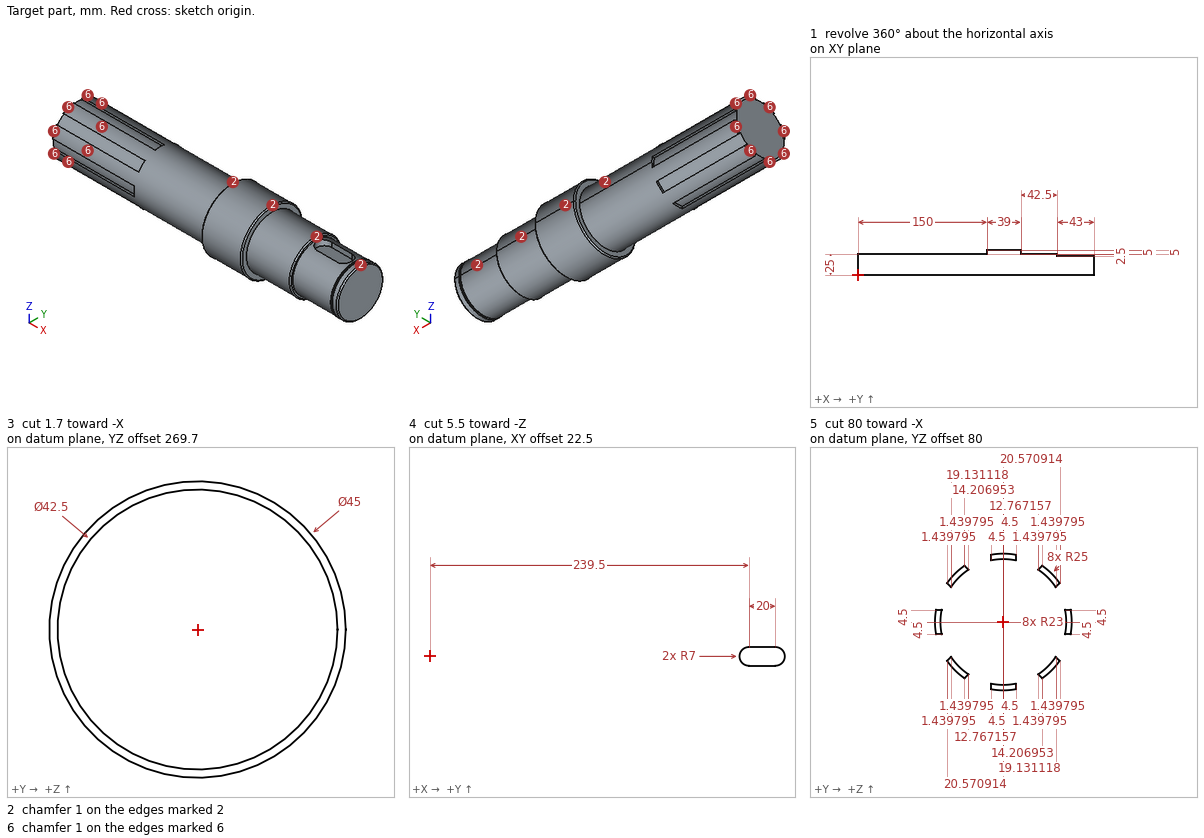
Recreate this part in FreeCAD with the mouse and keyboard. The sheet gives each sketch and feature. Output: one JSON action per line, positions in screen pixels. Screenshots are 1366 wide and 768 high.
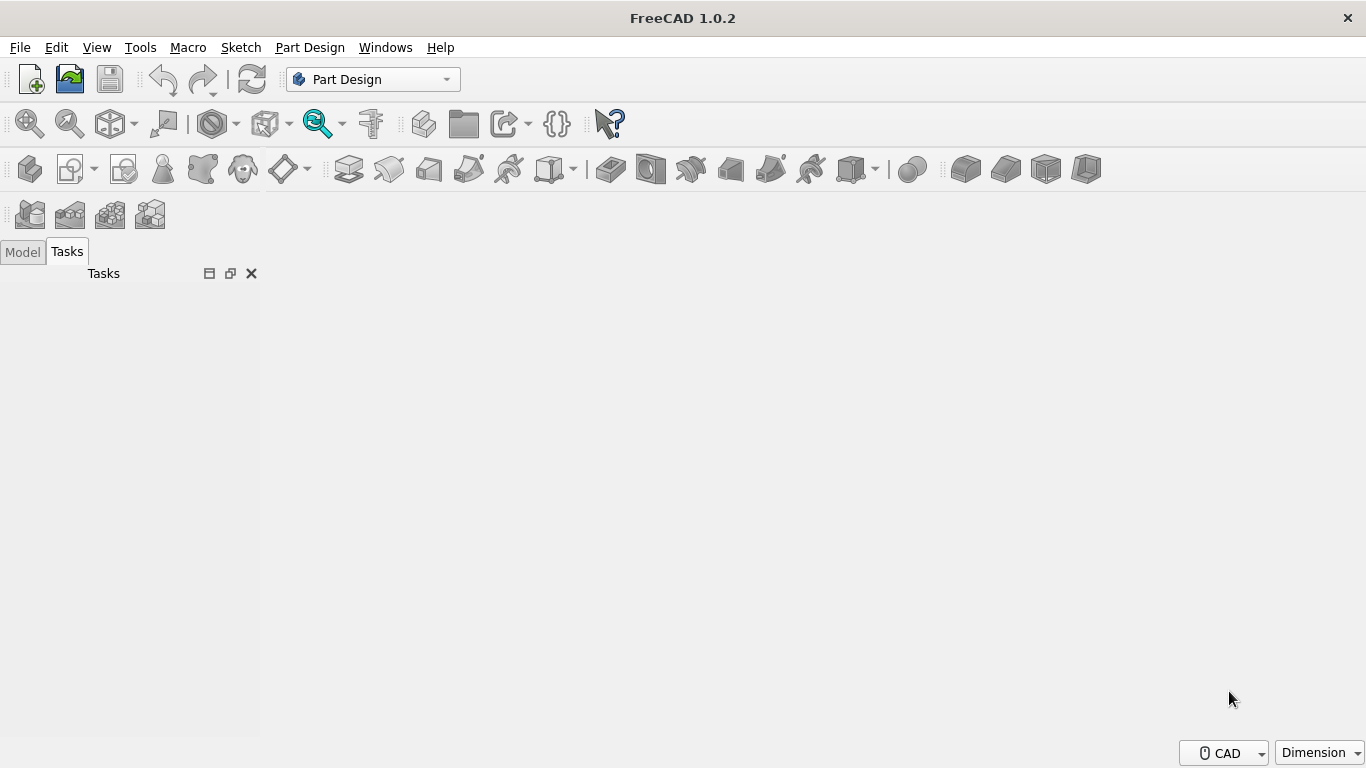
{"action": "left_click", "coordinate": [30, 80]}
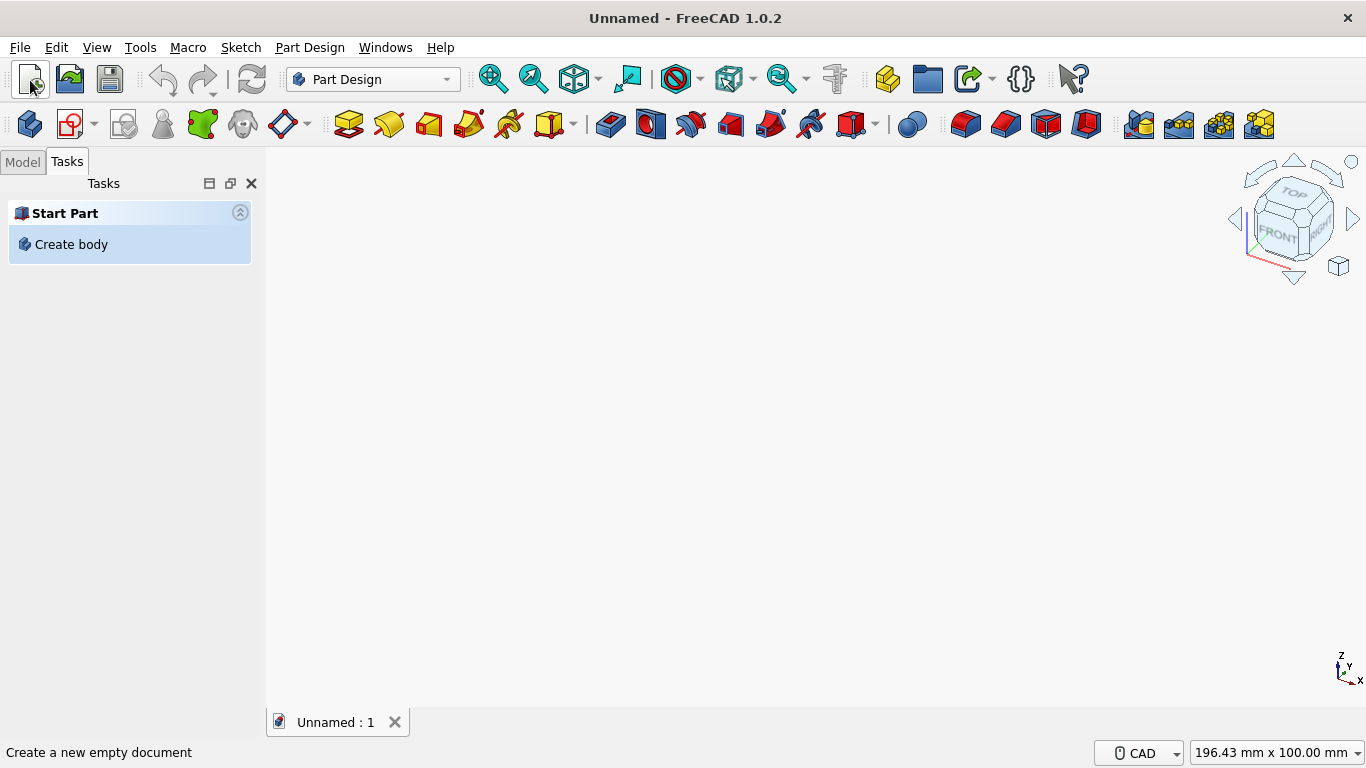
{"action": "left_click", "coordinate": [70, 124]}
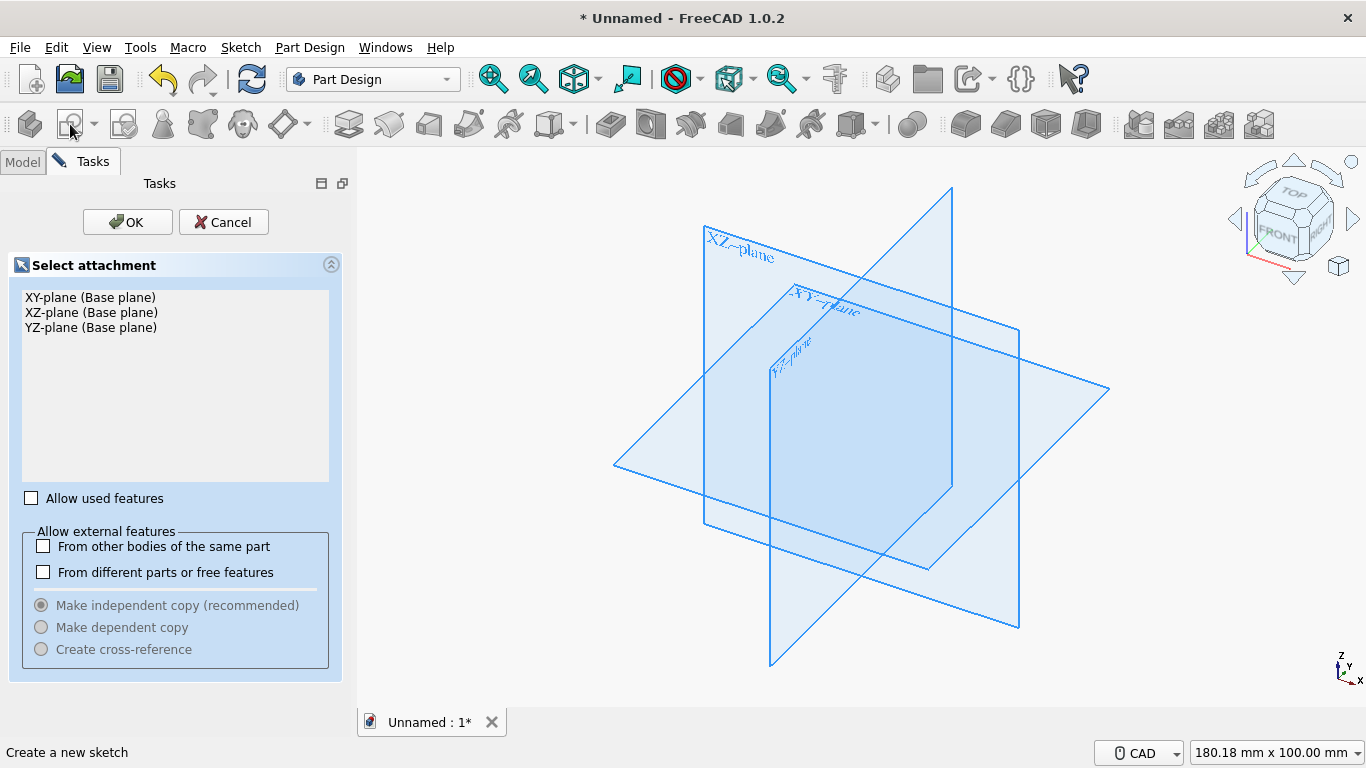
{"action": "left_click", "coordinate": [82, 298]}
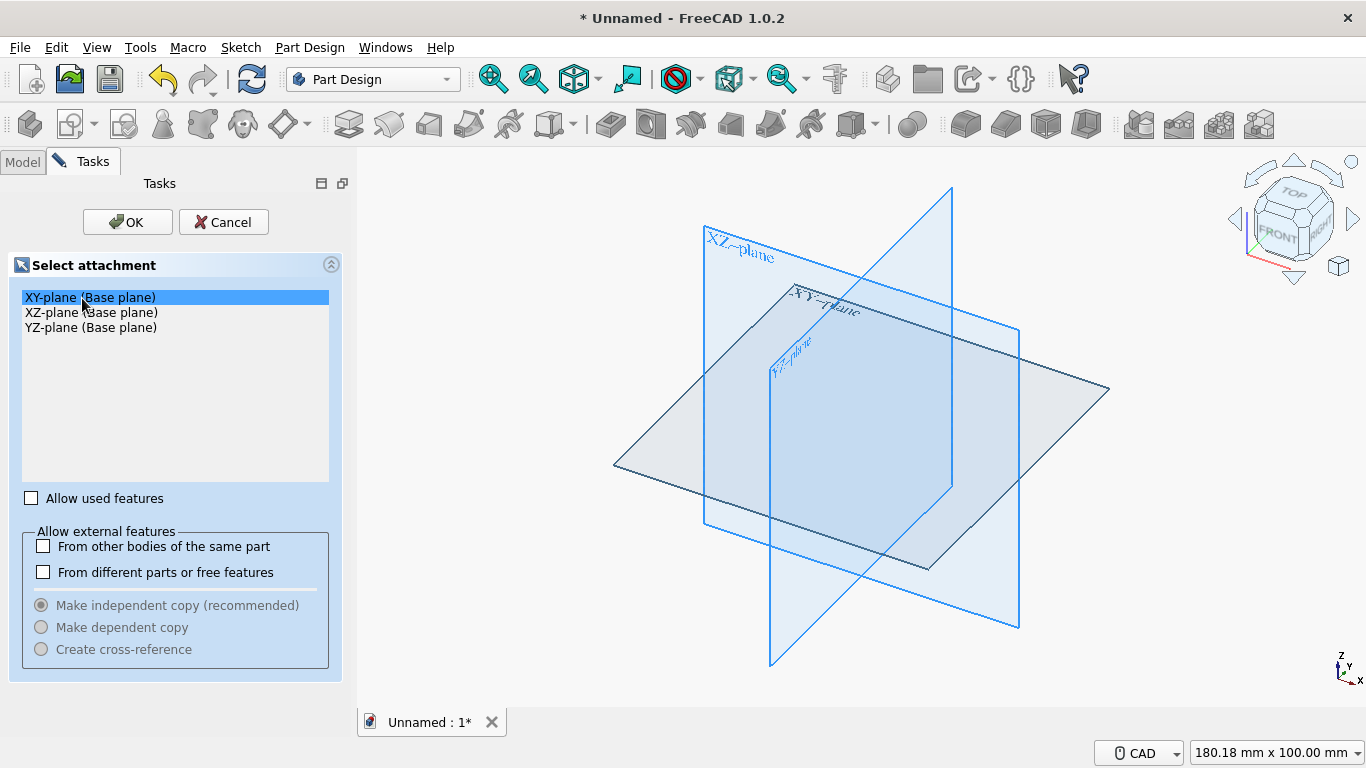
{"action": "left_click", "coordinate": [128, 222]}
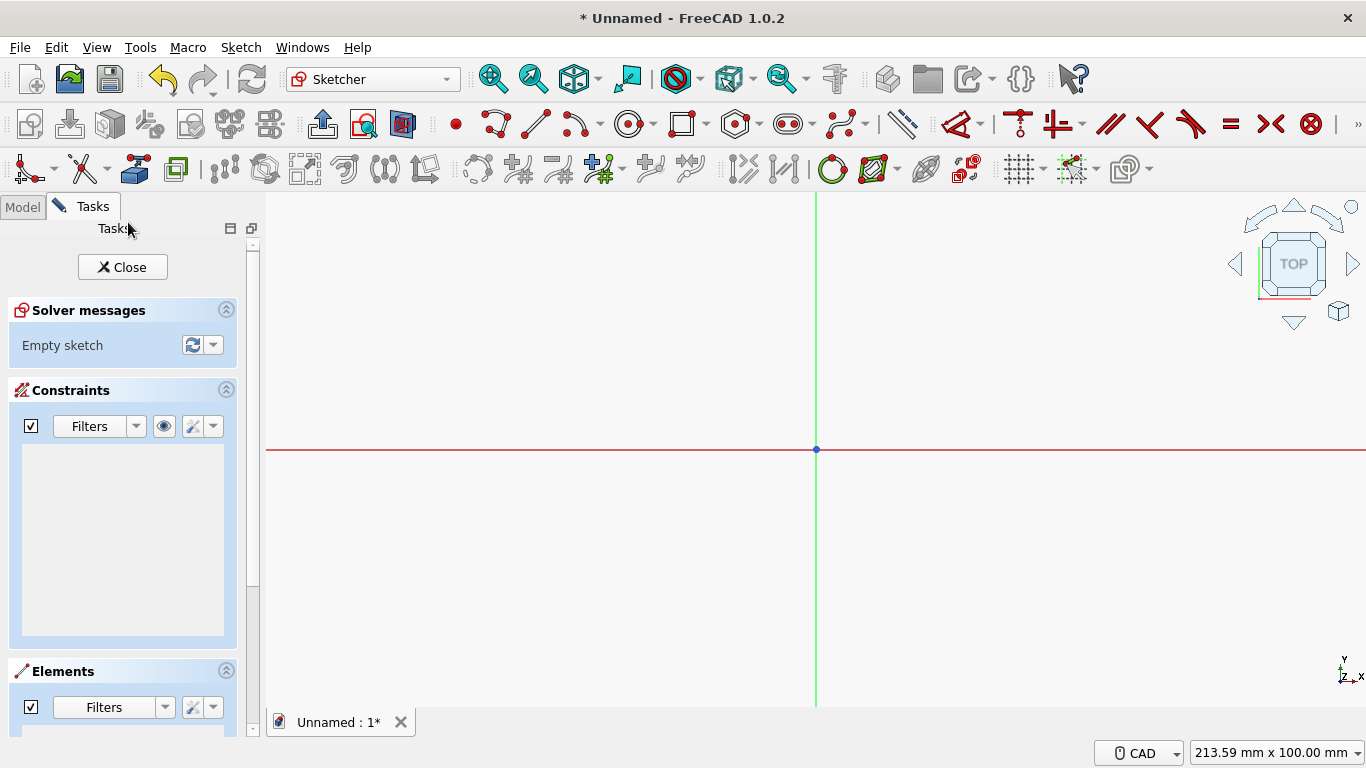
{"action": "scroll", "coordinate": [294, 513], "scroll_direction": "down", "scroll_amount": 4}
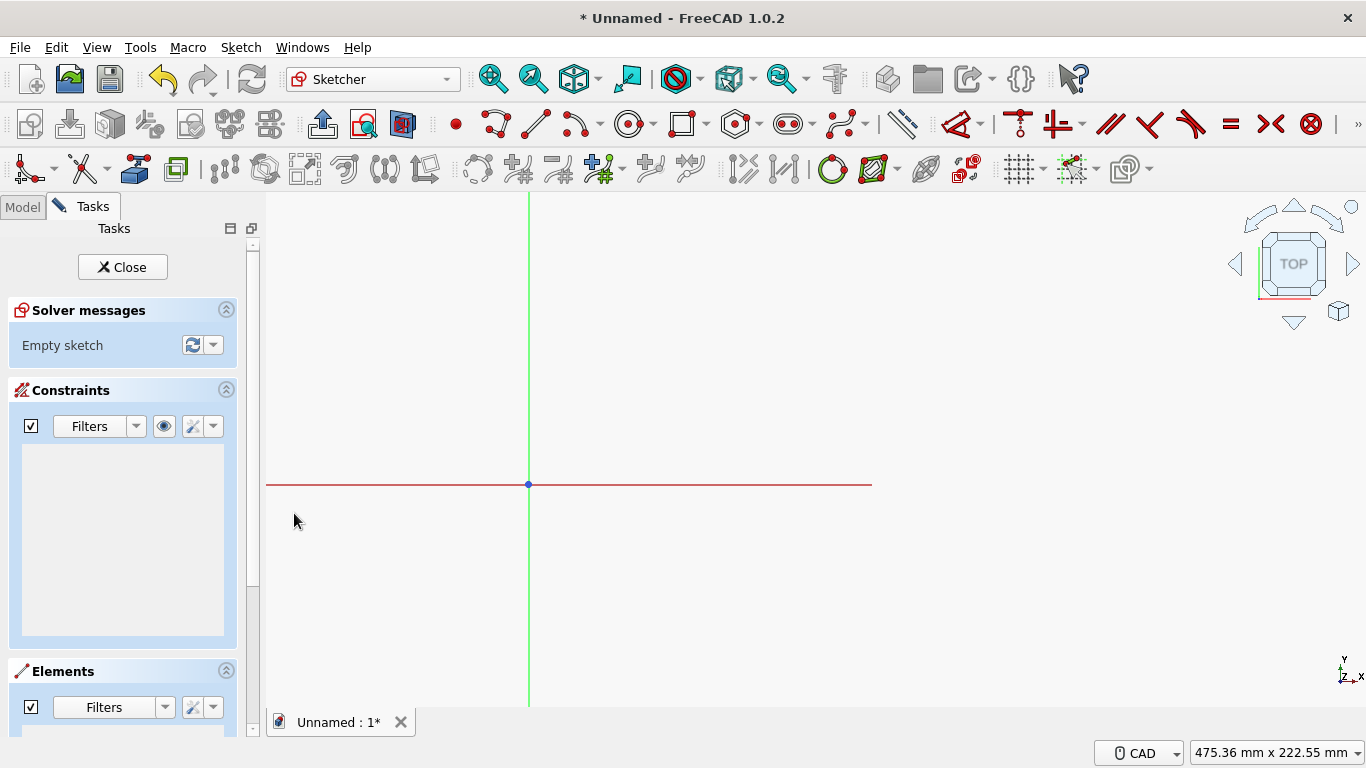
{"action": "left_click", "coordinate": [496, 124]}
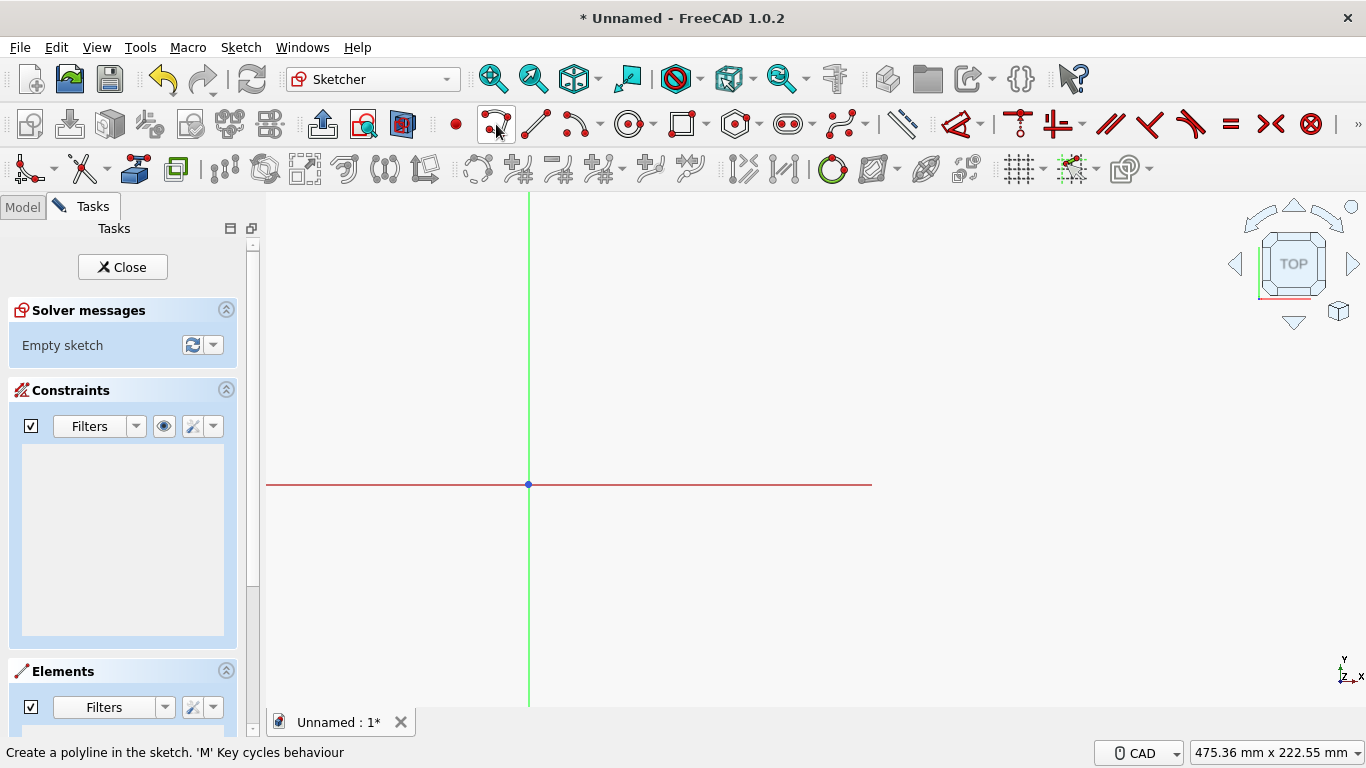
{"action": "left_click", "coordinate": [529, 485]}
{"action": "left_click", "coordinate": [1164, 476]}
{"action": "left_click", "coordinate": [1164, 433]}
{"action": "left_click", "coordinate": [1064, 433]}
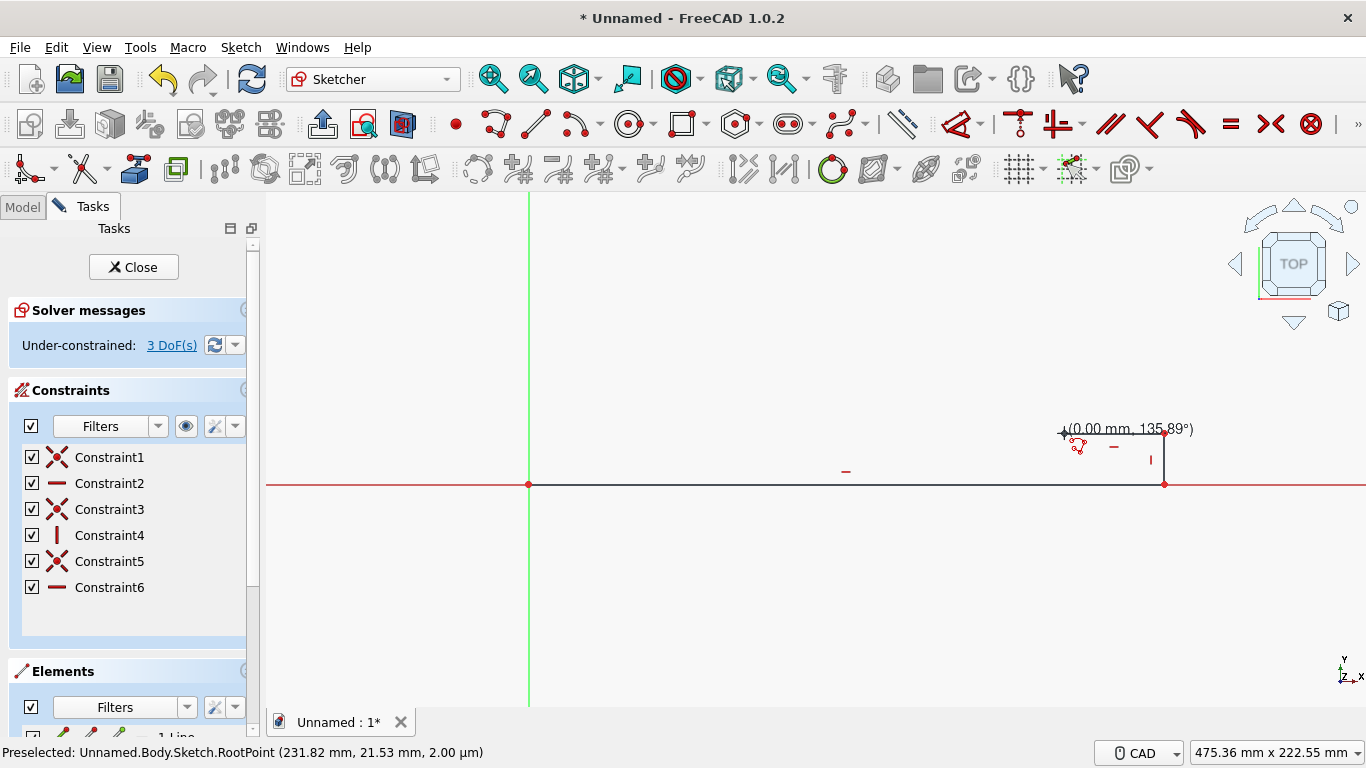
{"action": "scroll", "coordinate": [1064, 427], "scroll_direction": "up", "scroll_amount": 6}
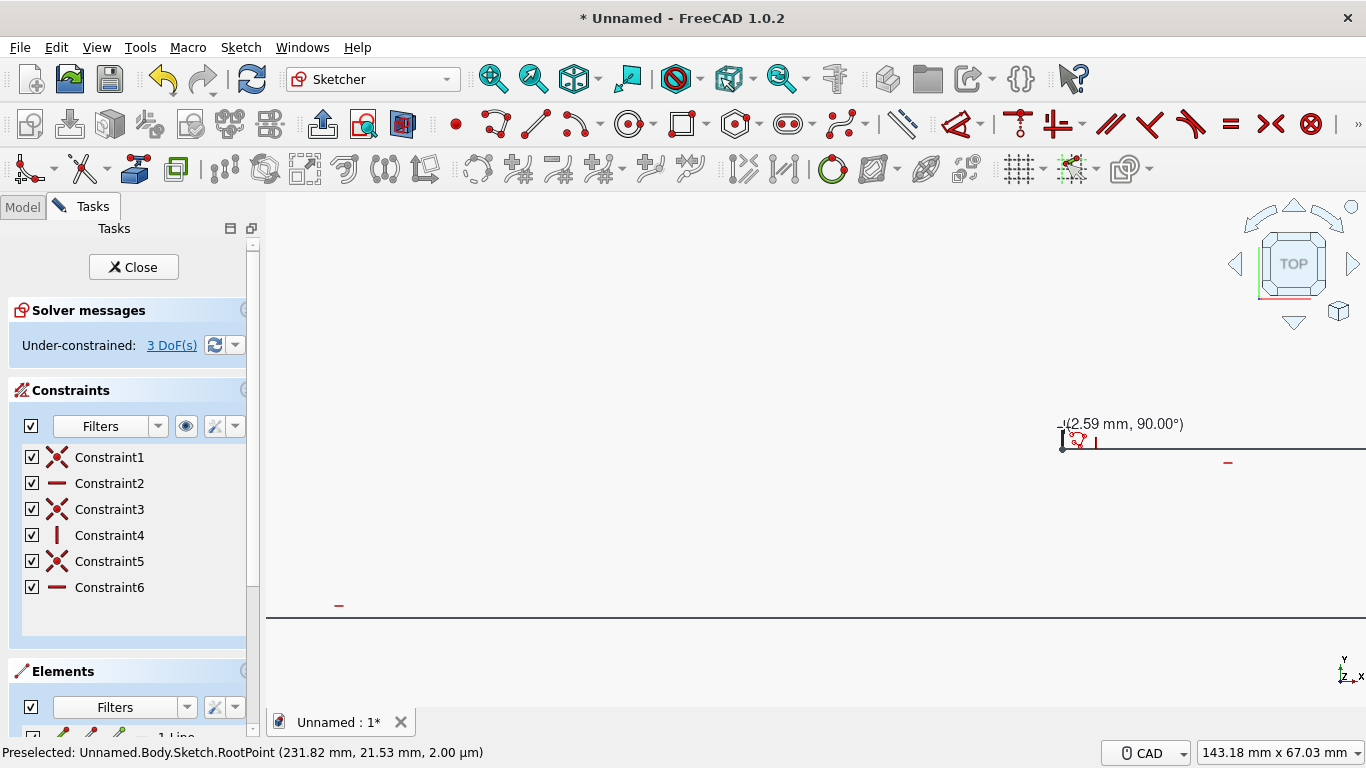
{"action": "left_click", "coordinate": [1062, 426]}
{"action": "left_click", "coordinate": [737, 426]}
{"action": "left_click", "coordinate": [737, 387]}
{"action": "left_click", "coordinate": [437, 387]}
{"action": "left_click", "coordinate": [437, 426]}